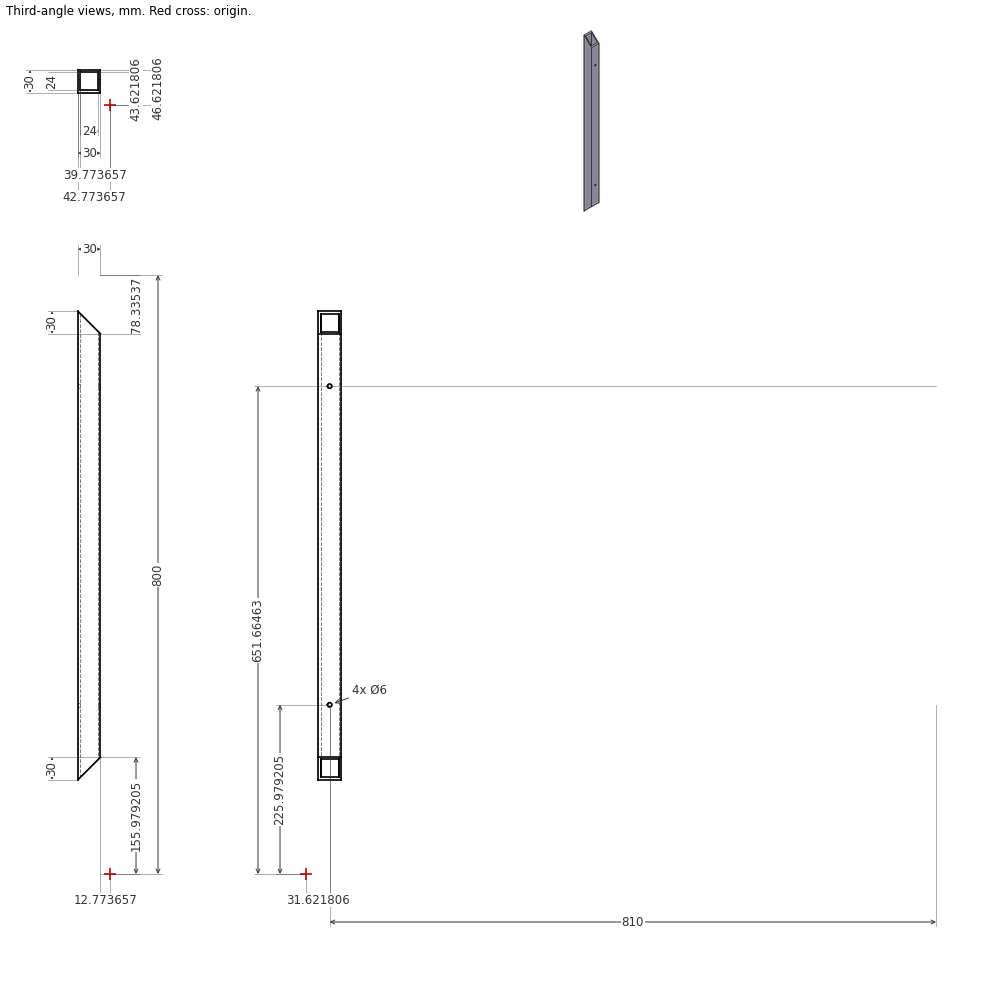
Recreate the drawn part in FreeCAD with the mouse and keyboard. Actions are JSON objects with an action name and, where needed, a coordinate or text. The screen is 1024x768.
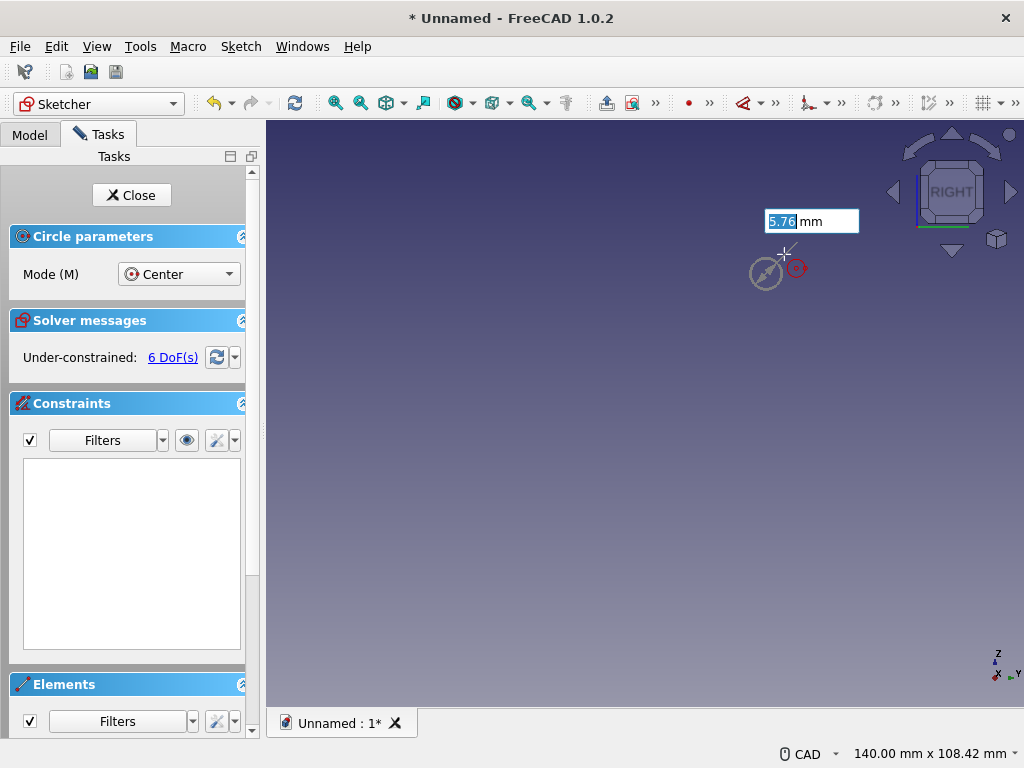
{"action": "left_click", "coordinate": [775, 247]}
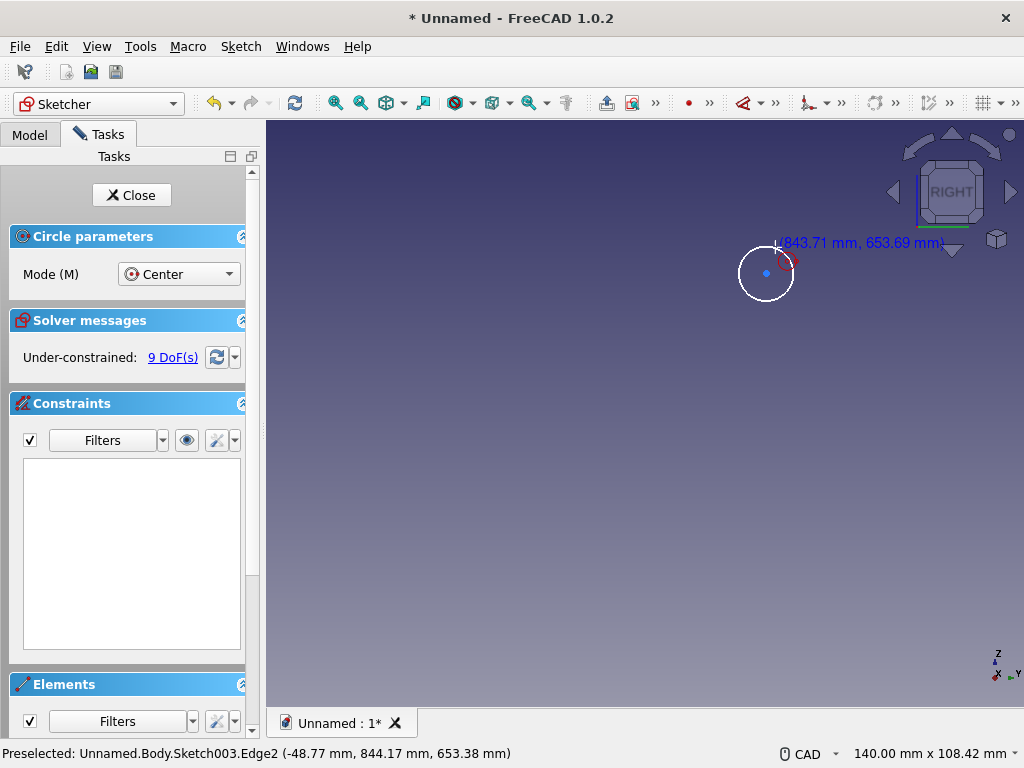
{"action": "scroll", "coordinate": [784, 254], "scroll_direction": "down", "scroll_amount": 12}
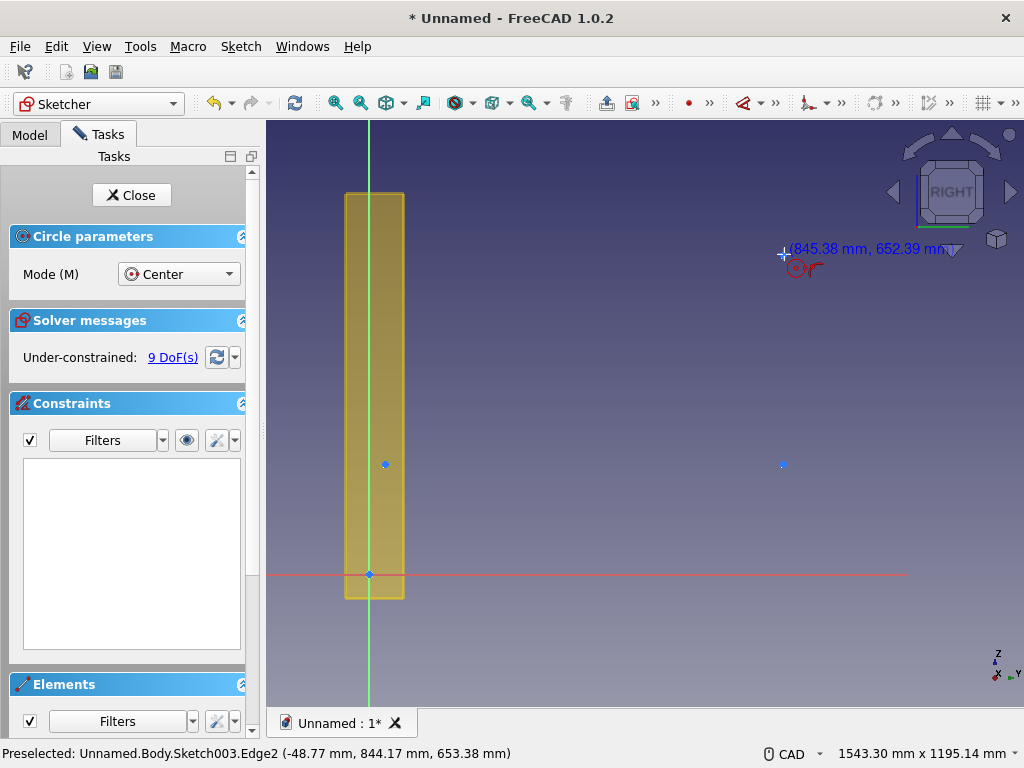
{"action": "scroll", "coordinate": [385, 255], "scroll_direction": "up", "scroll_amount": 14}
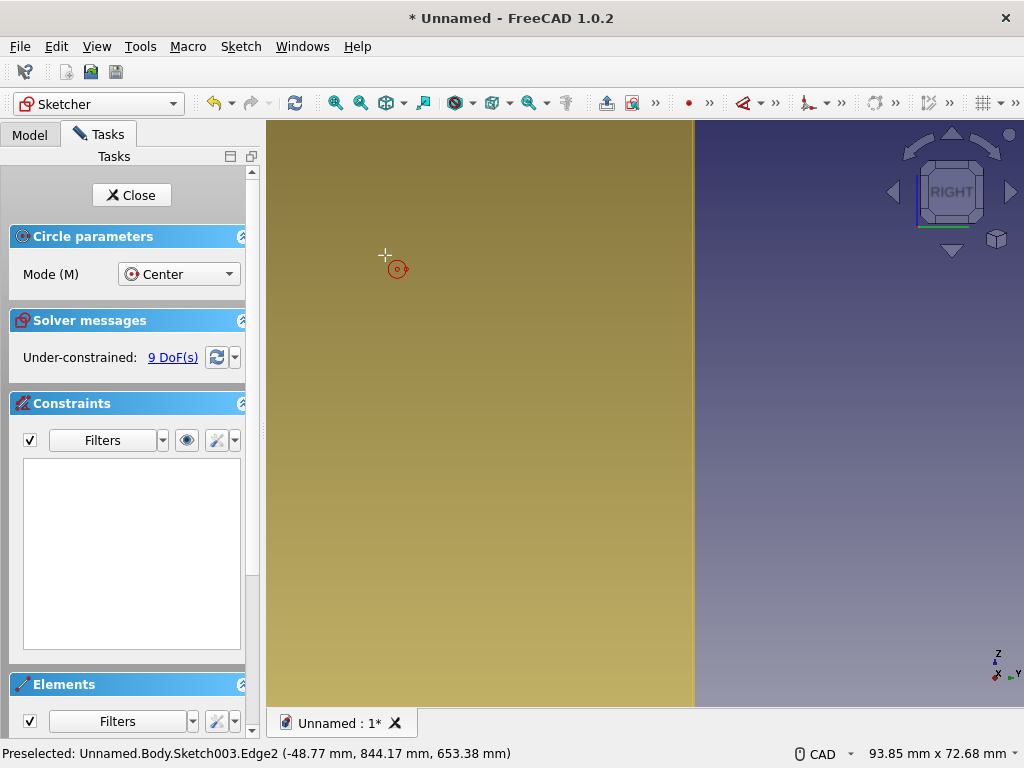
{"action": "scroll", "coordinate": [385, 255], "scroll_direction": "down", "scroll_amount": 14}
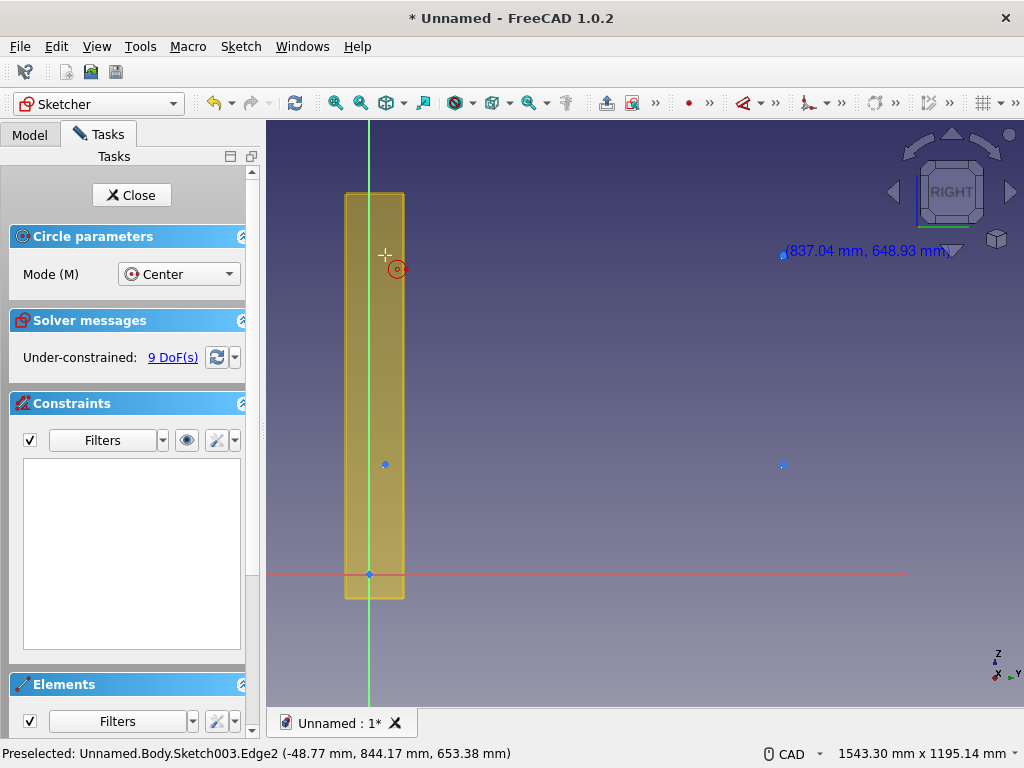
{"action": "left_click", "coordinate": [385, 255]}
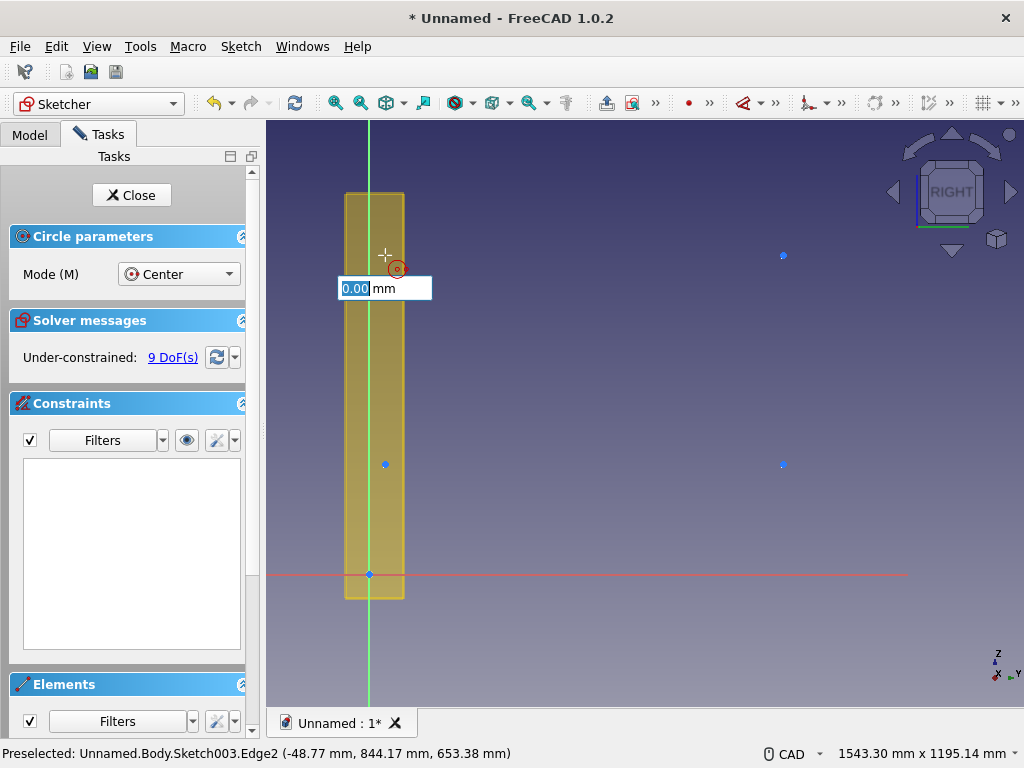
{"action": "scroll", "coordinate": [386, 254], "scroll_direction": "up", "scroll_amount": 12}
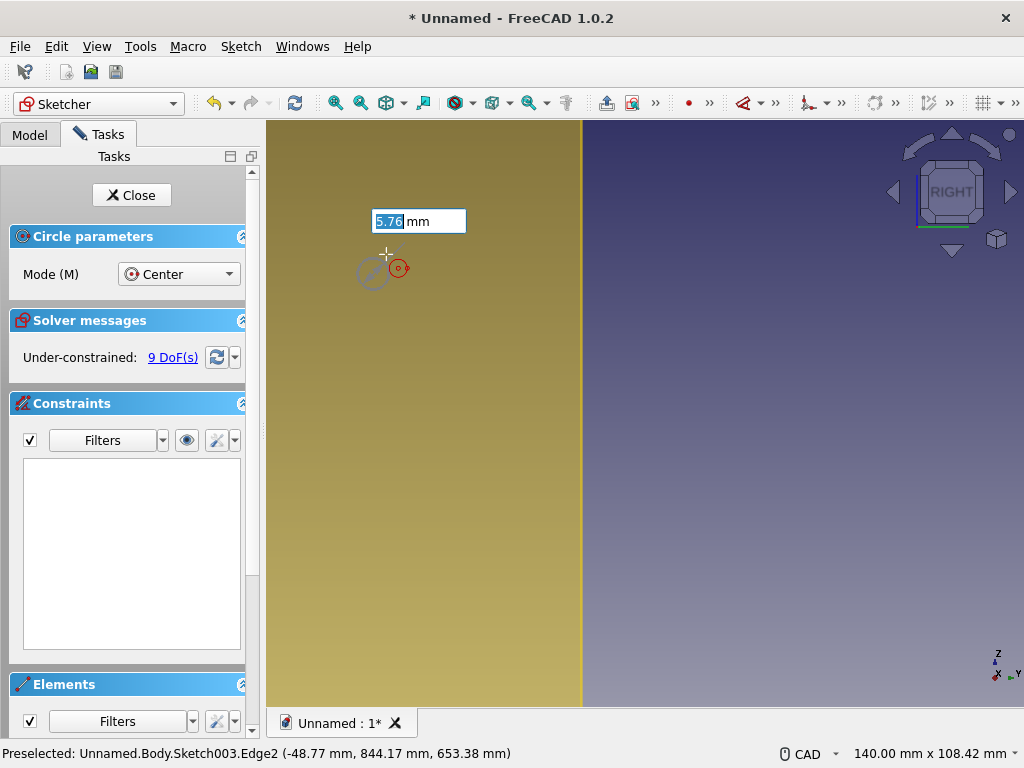
{"action": "left_click", "coordinate": [384, 247]}
{"action": "key", "text": "Escape"}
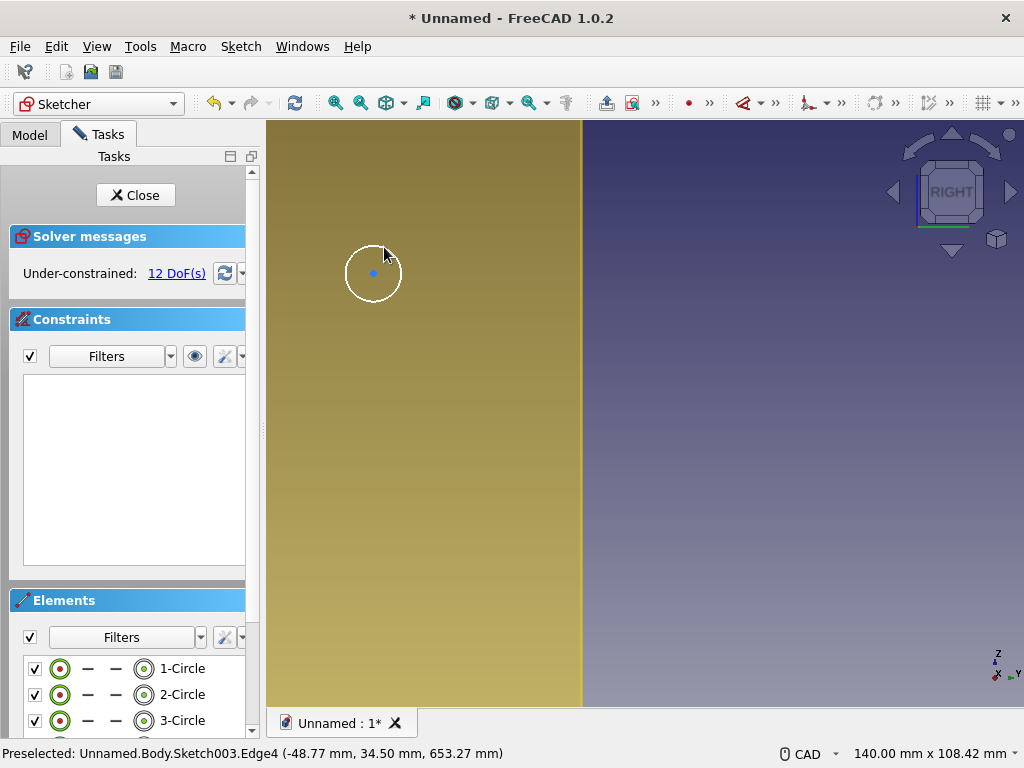
{"action": "scroll", "coordinate": [386, 254], "scroll_direction": "down", "scroll_amount": 12}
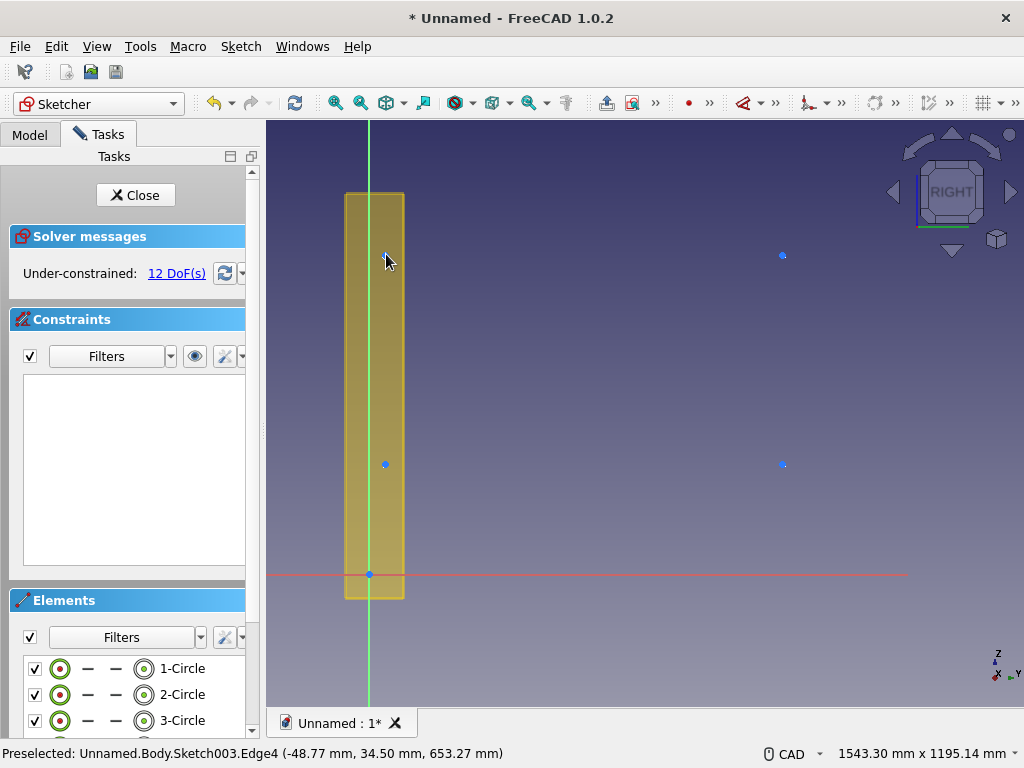
{"action": "scroll", "coordinate": [387, 463], "scroll_direction": "up", "scroll_amount": 9}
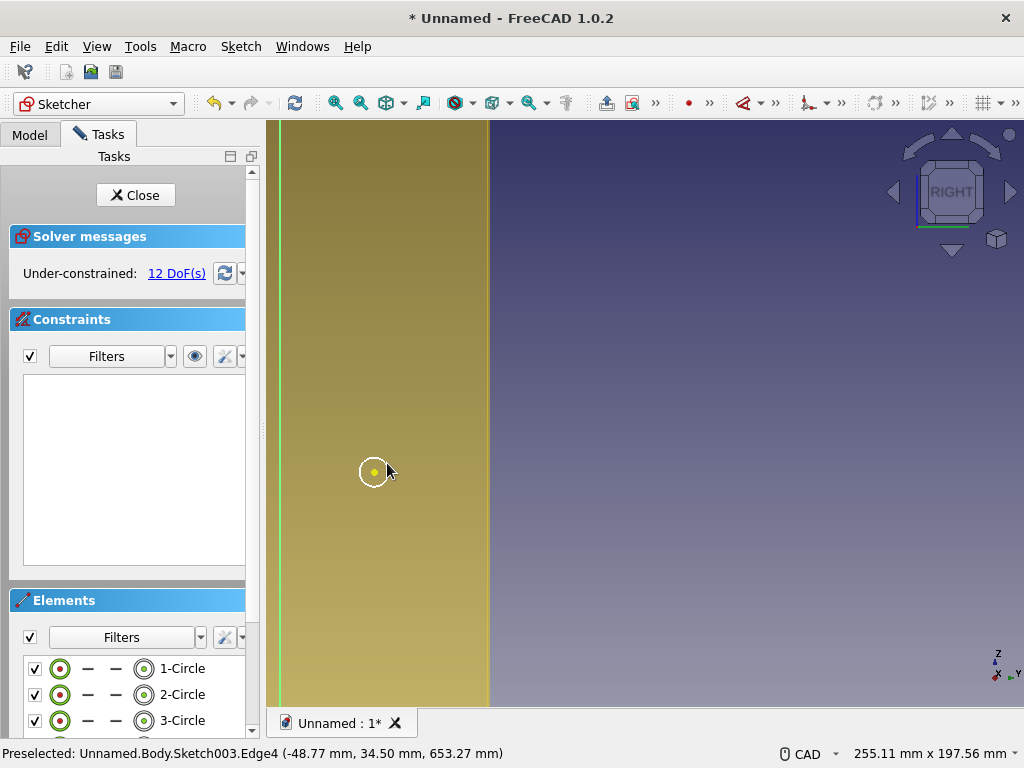
{"action": "left_click", "coordinate": [384, 462]}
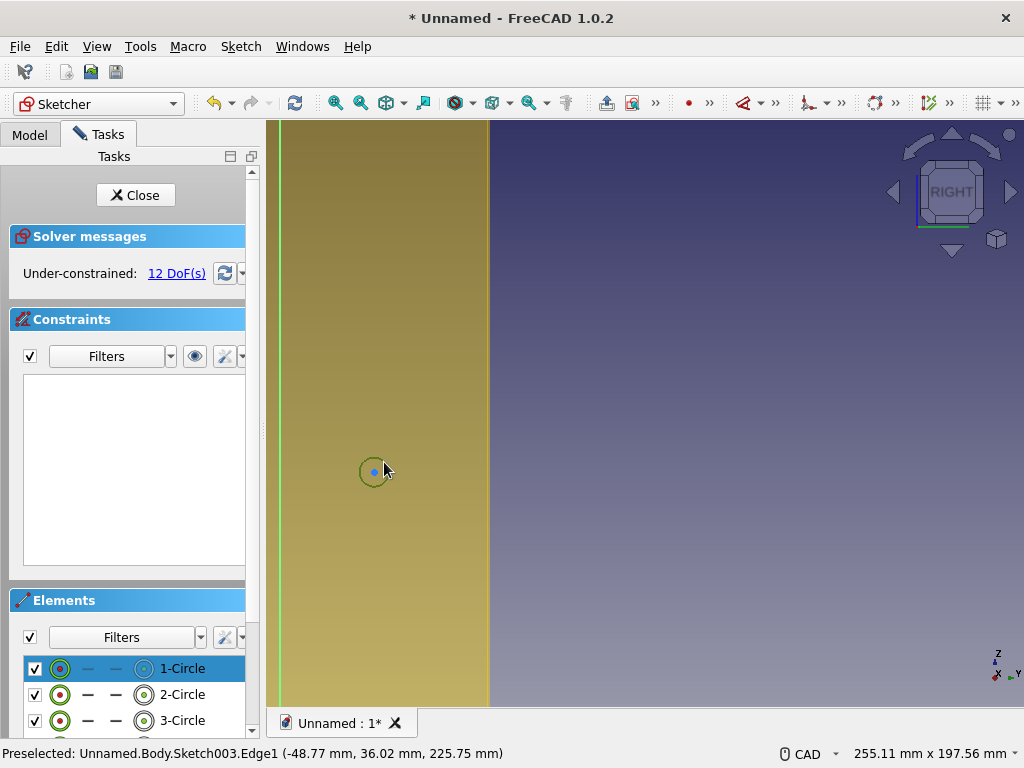
{"action": "scroll", "coordinate": [387, 463], "scroll_direction": "down", "scroll_amount": 9}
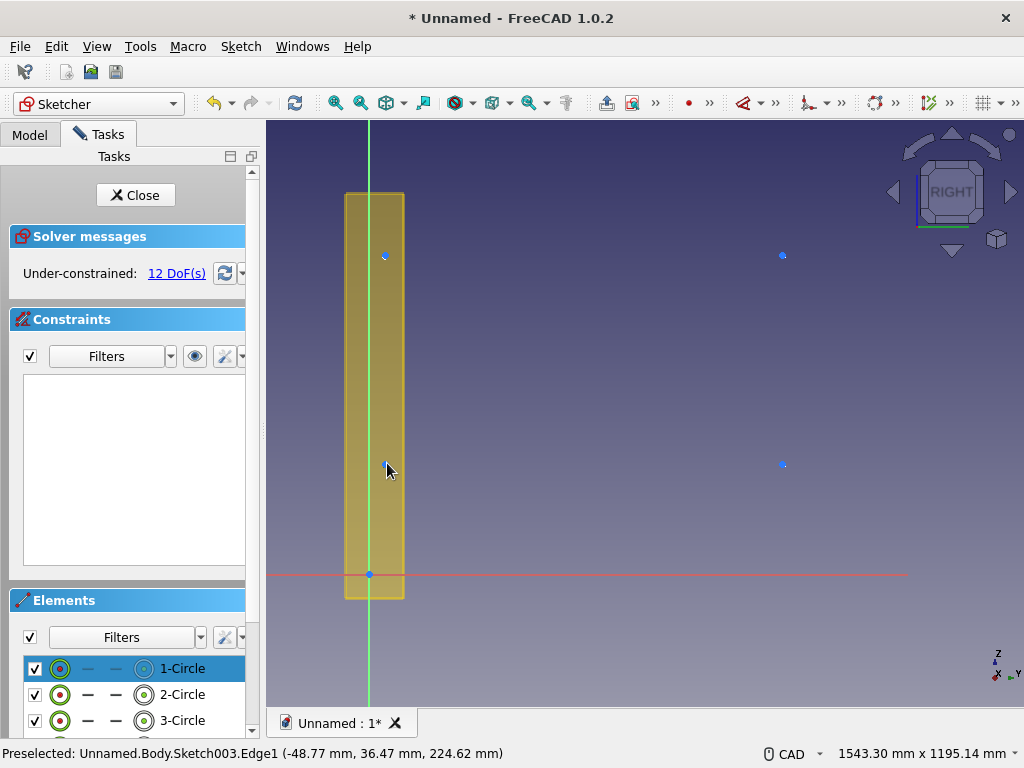
{"action": "scroll", "coordinate": [785, 463], "scroll_direction": "up", "scroll_amount": 9}